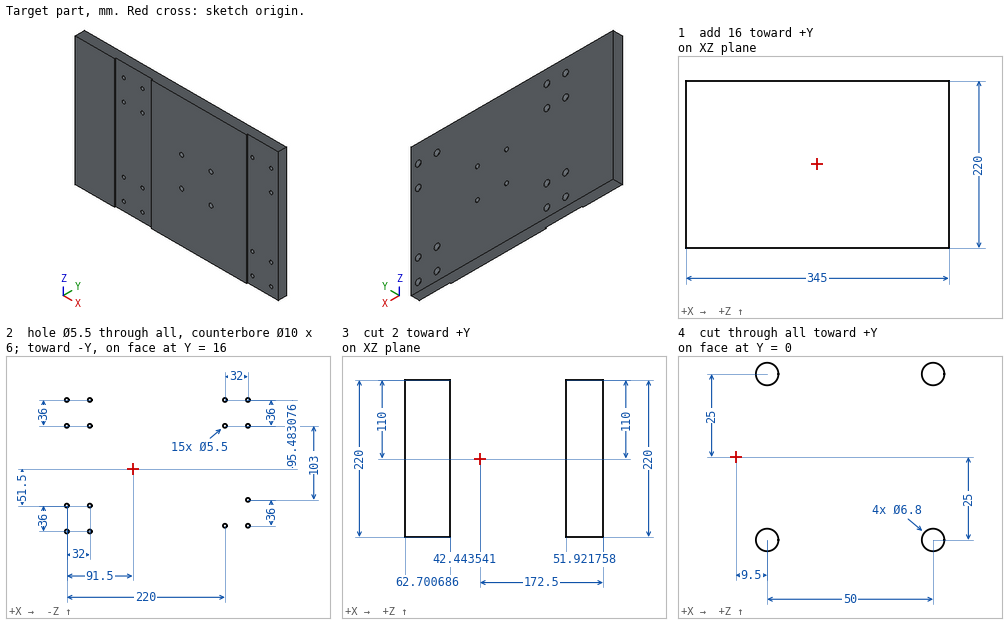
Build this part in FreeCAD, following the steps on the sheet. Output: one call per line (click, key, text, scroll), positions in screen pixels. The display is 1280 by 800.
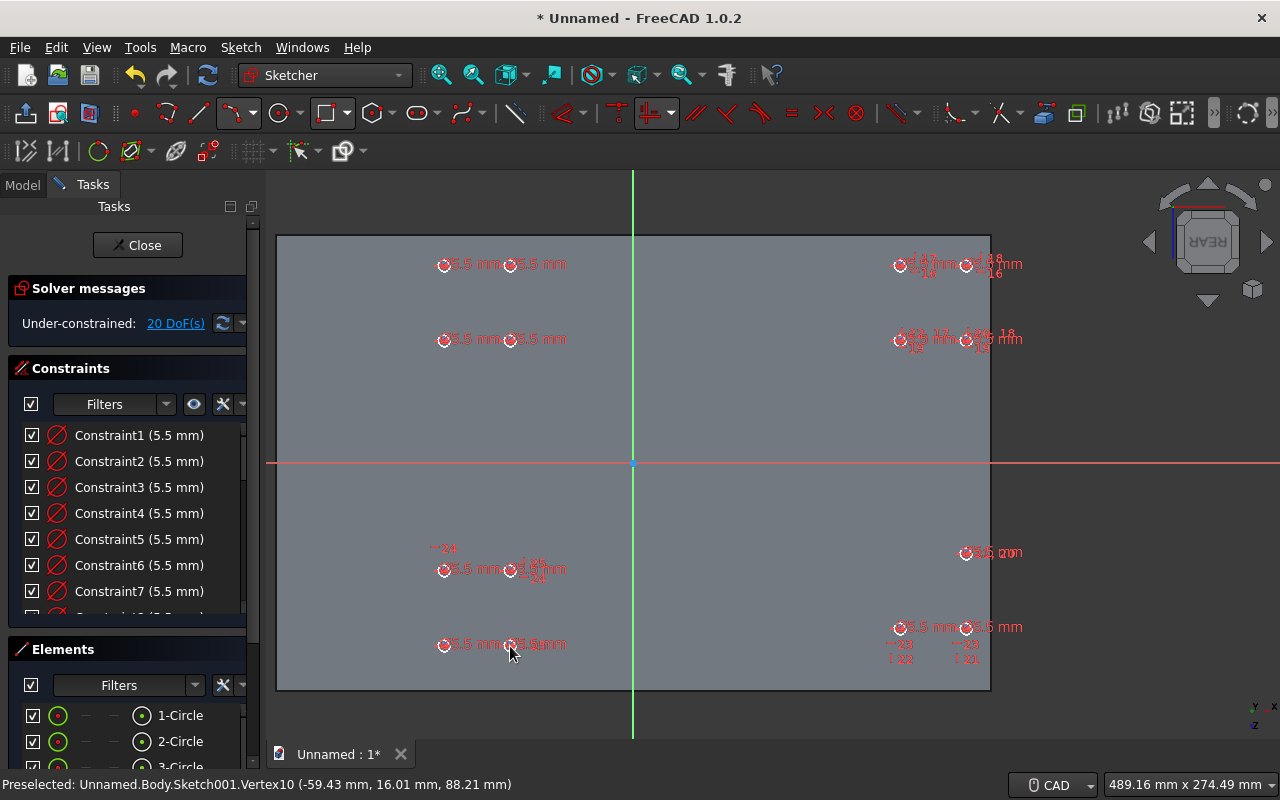
click(444, 571)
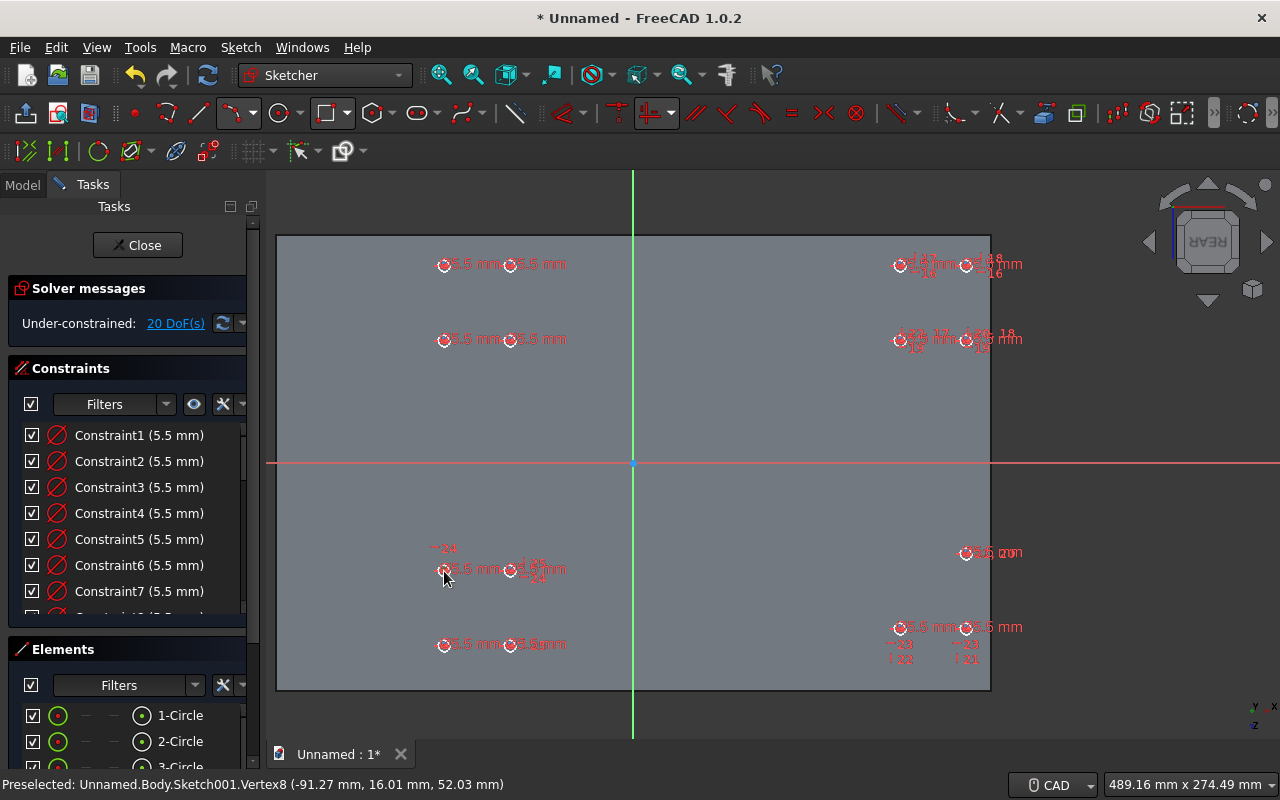
click(444, 646)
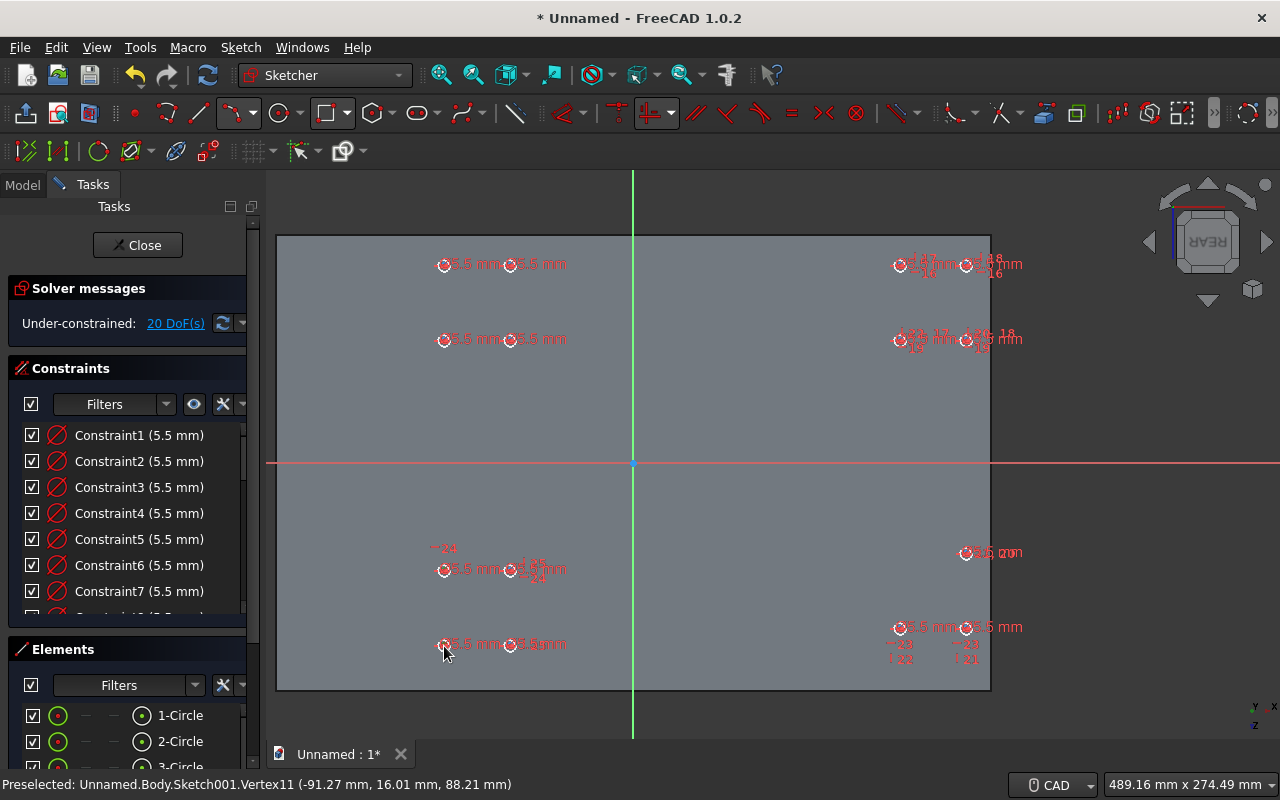
key(v)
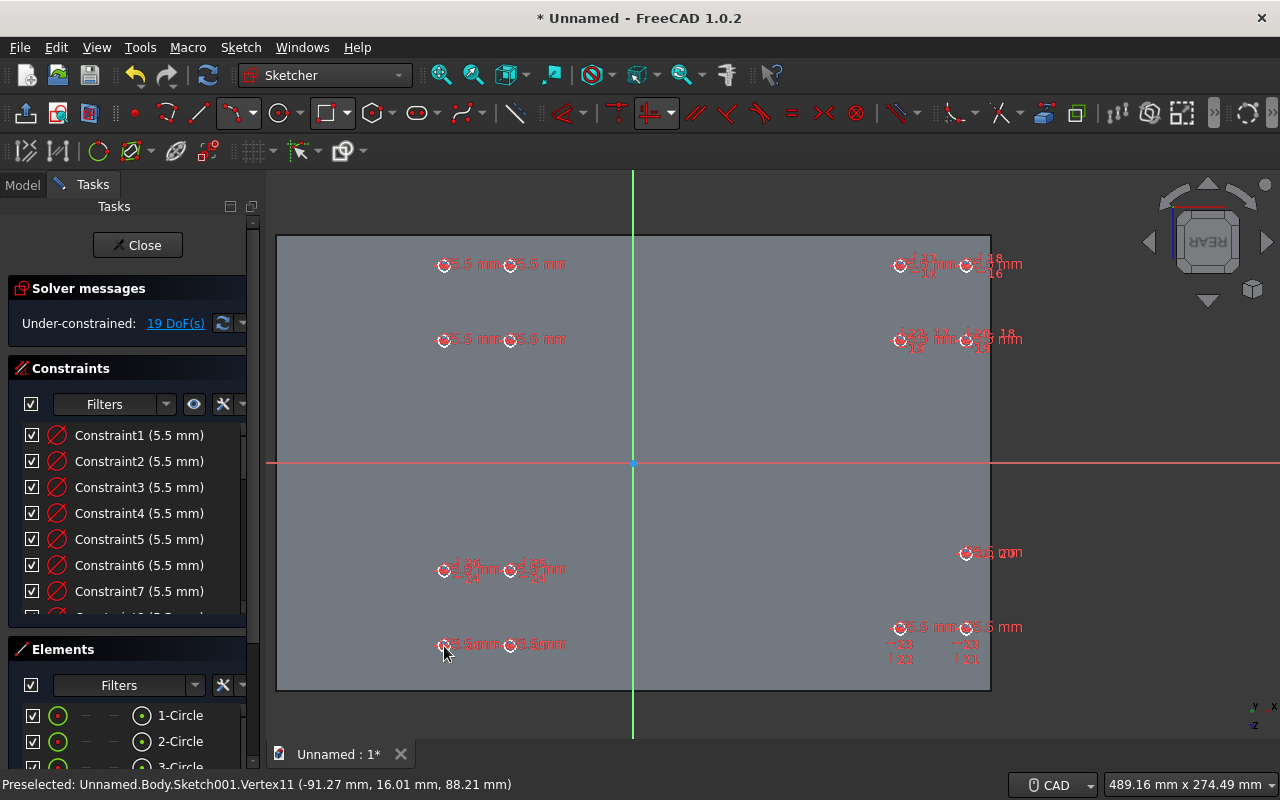
click(510, 646)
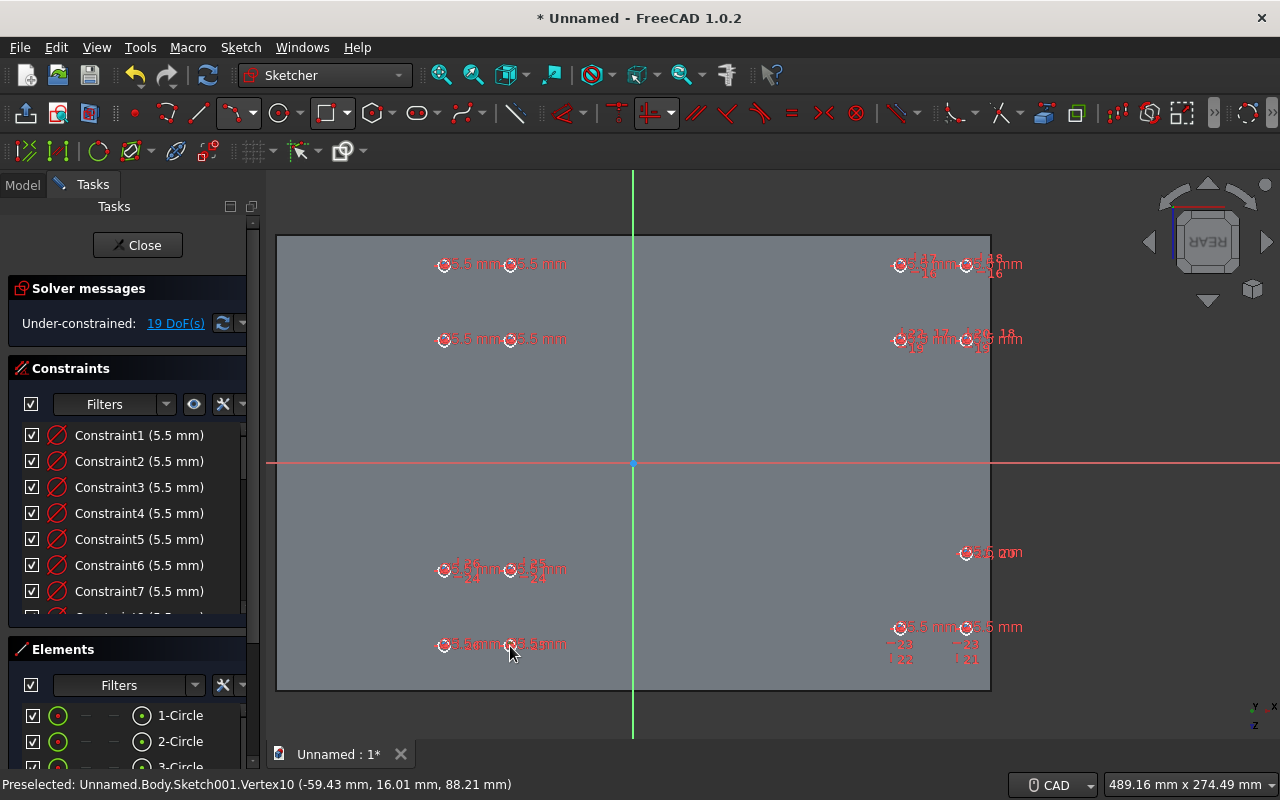
click(444, 646)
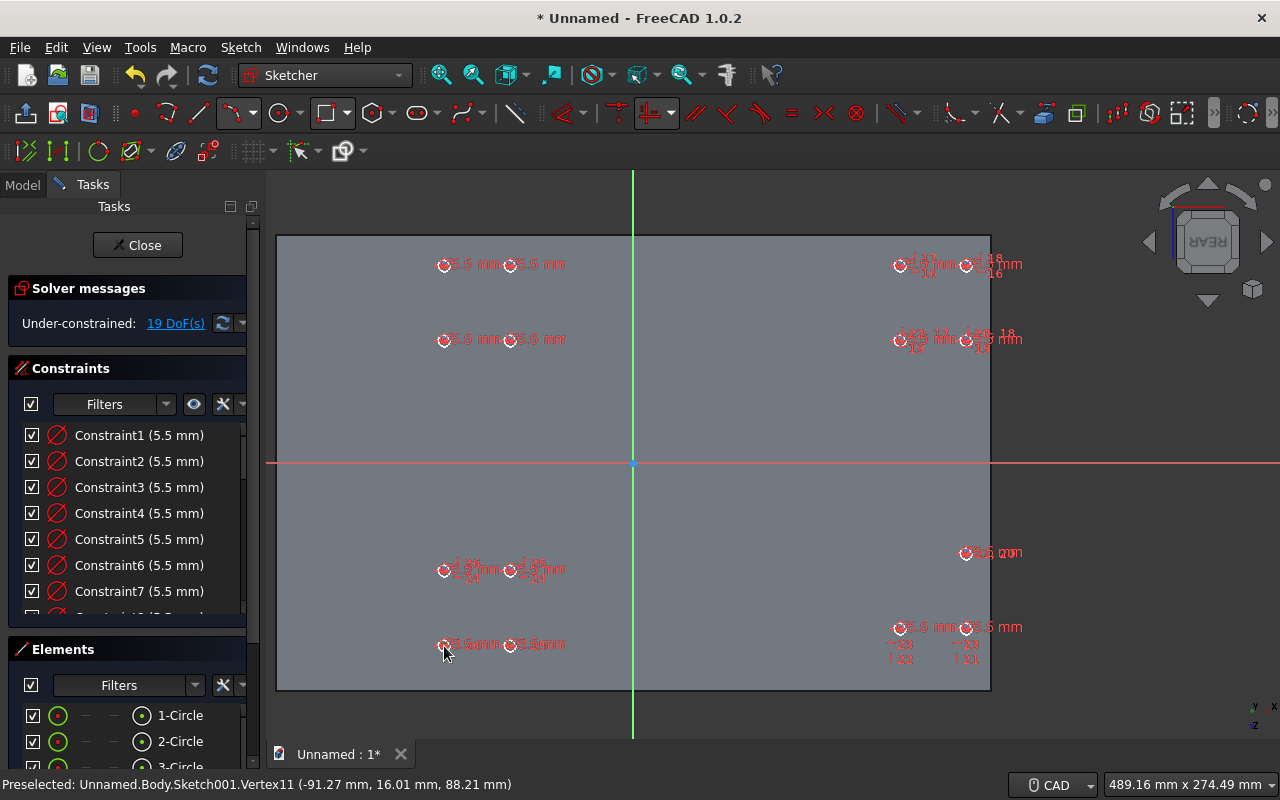
key(h)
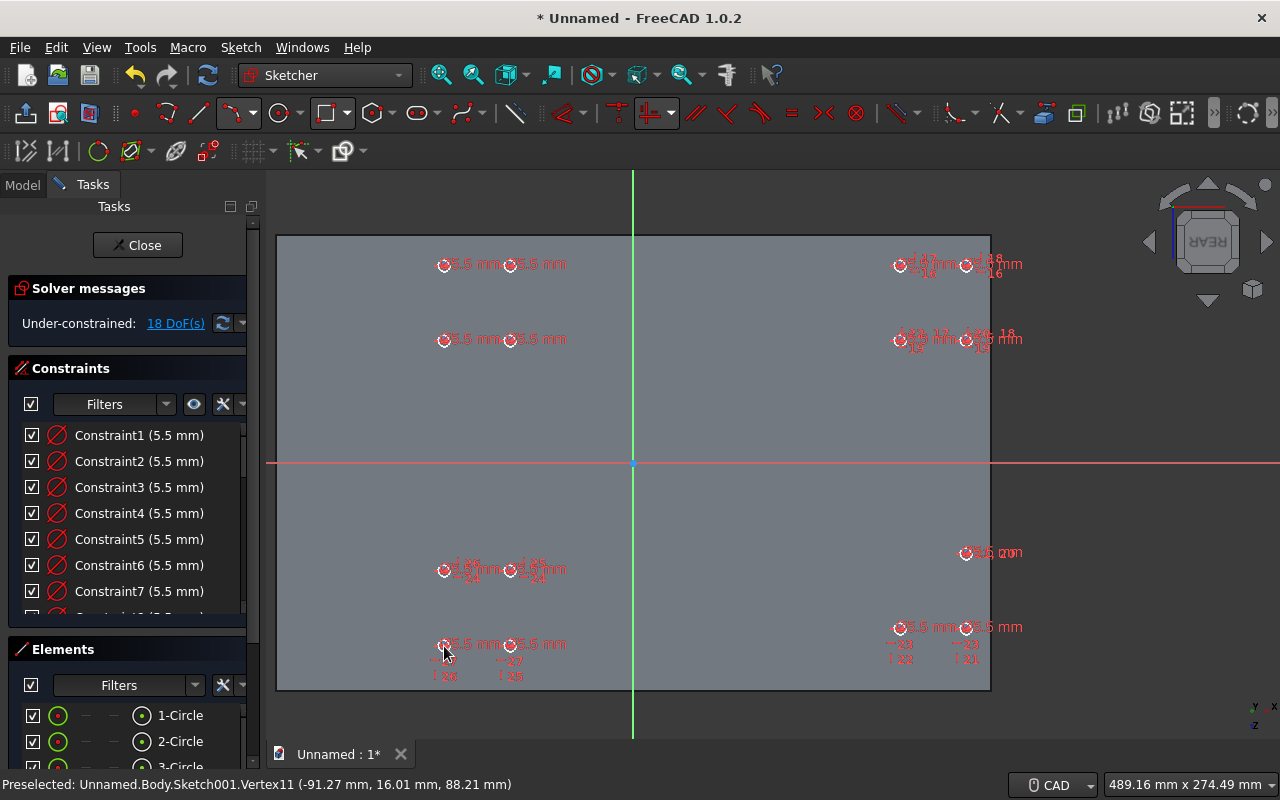
click(444, 571)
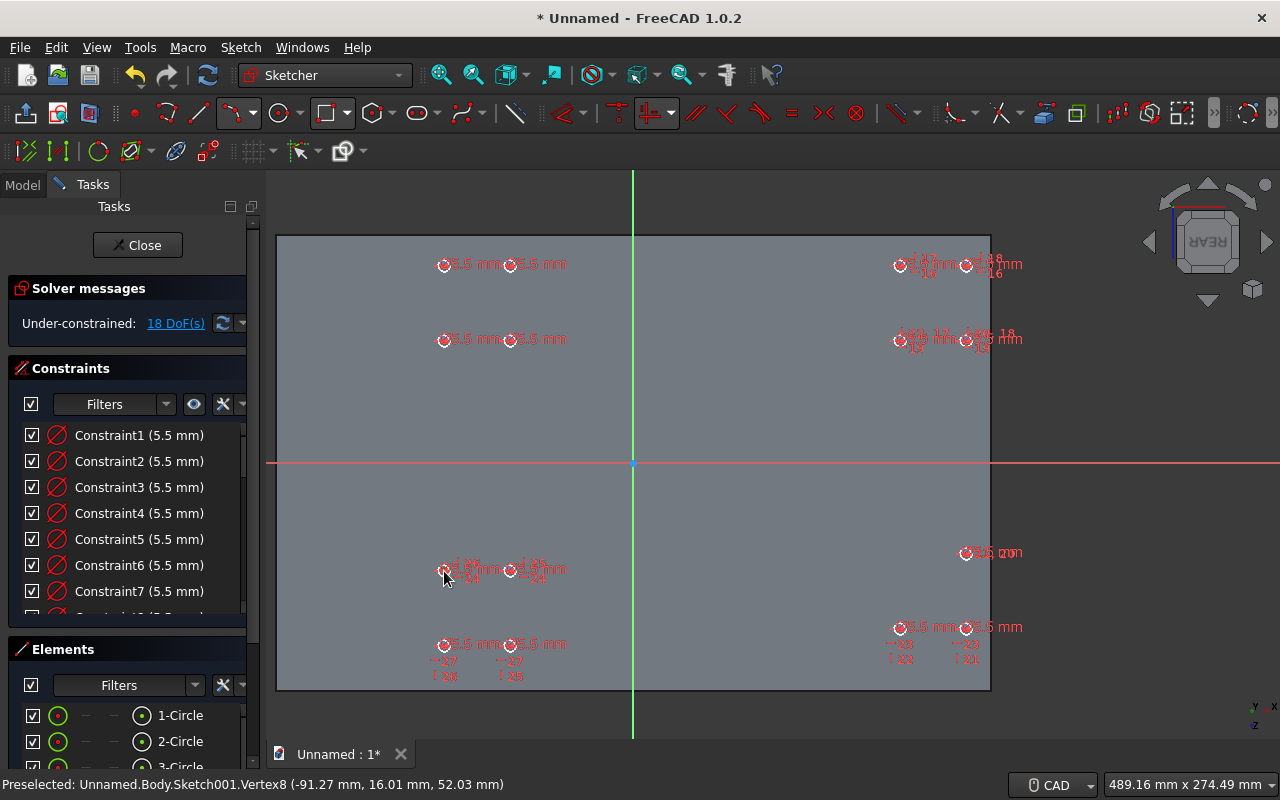
click(444, 341)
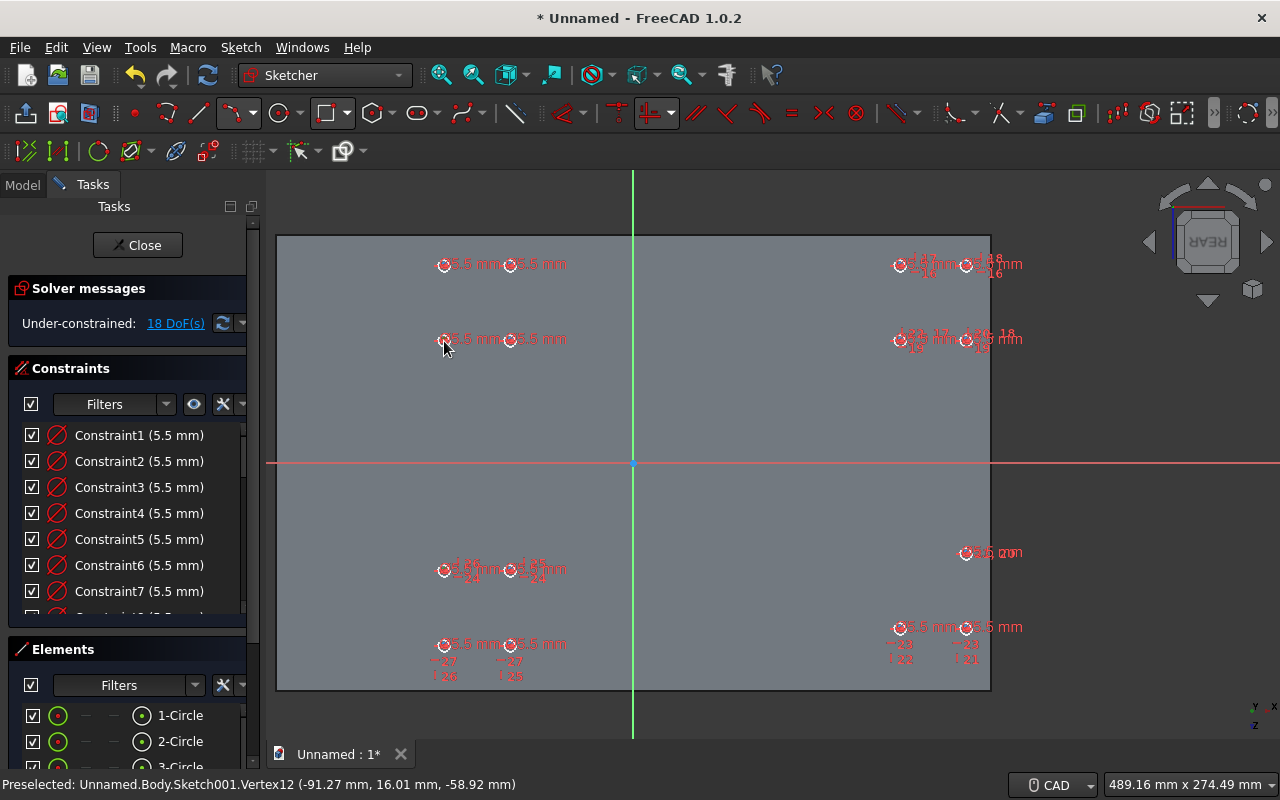
click(674, 114)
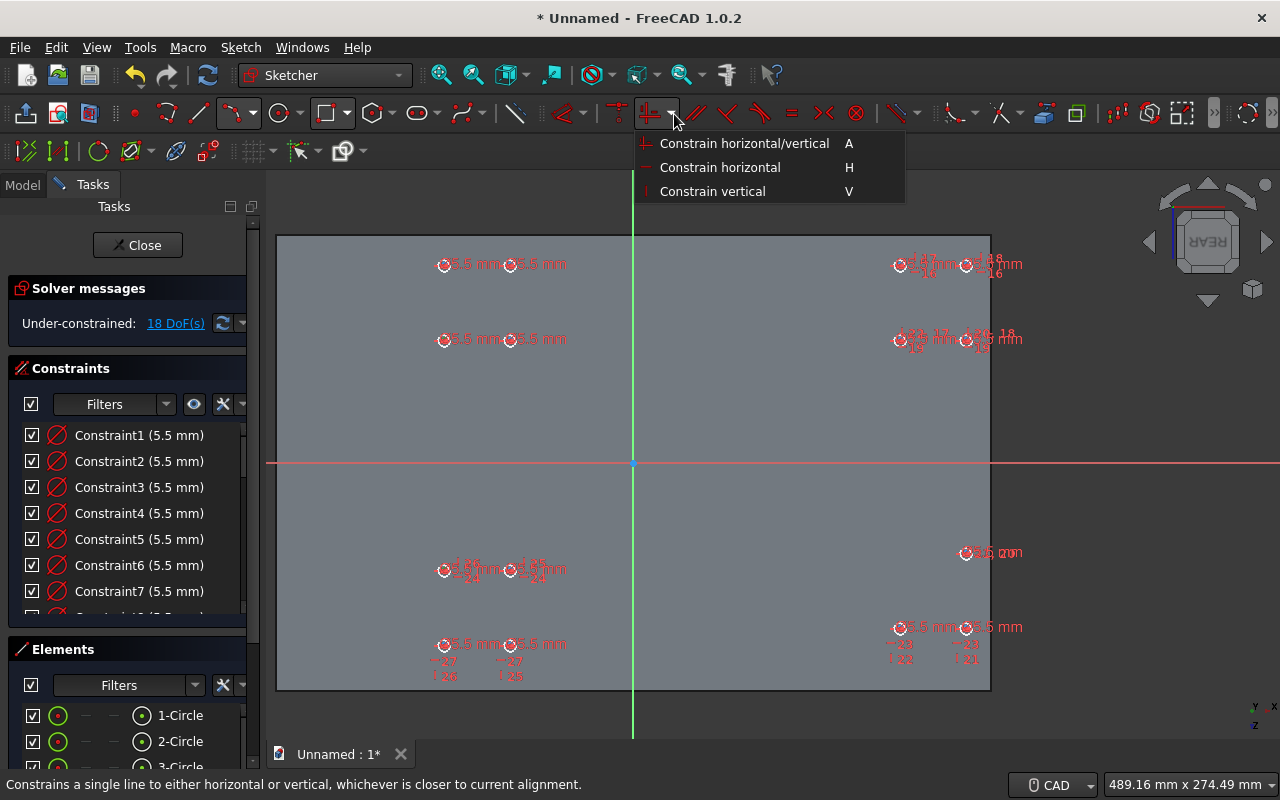
click(770, 191)